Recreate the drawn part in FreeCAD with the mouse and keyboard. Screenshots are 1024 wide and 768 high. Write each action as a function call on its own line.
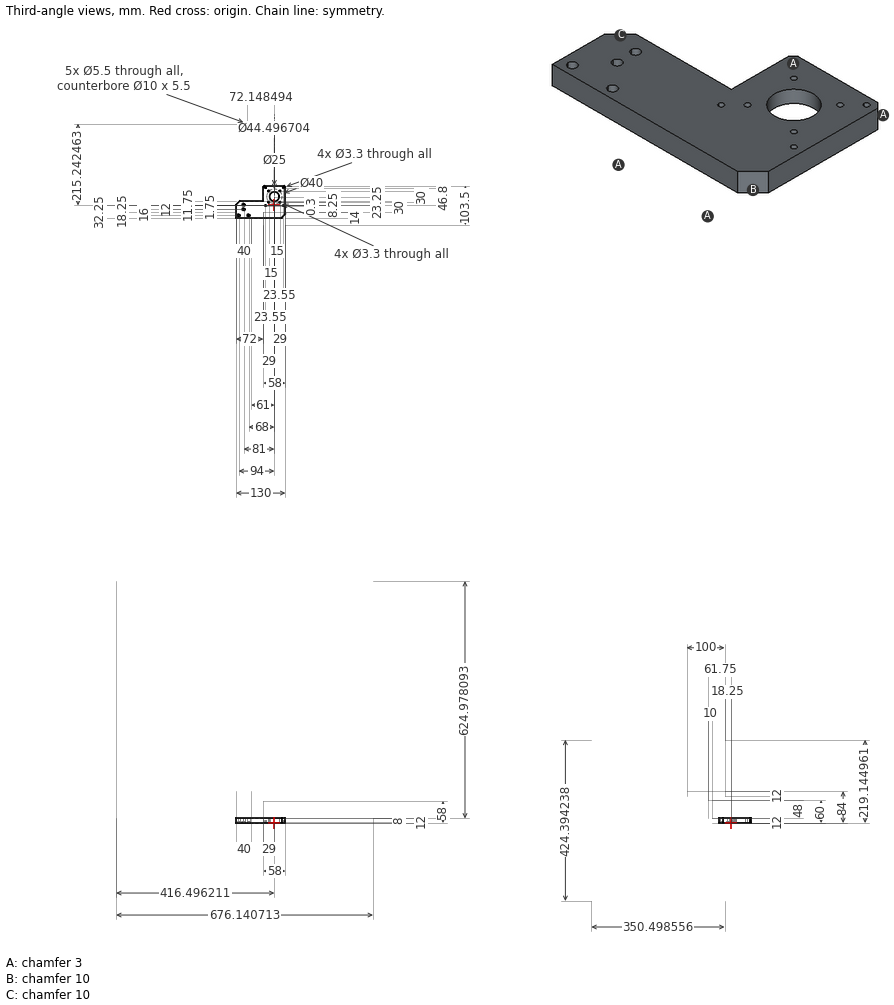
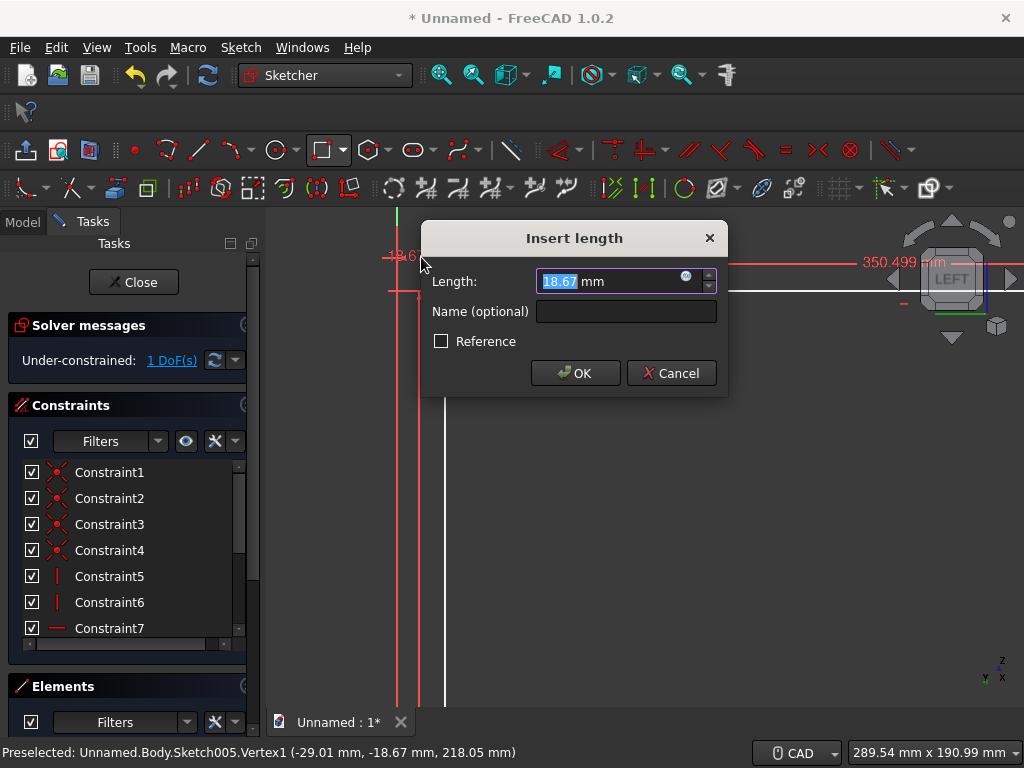
text(18.25)
key(Return)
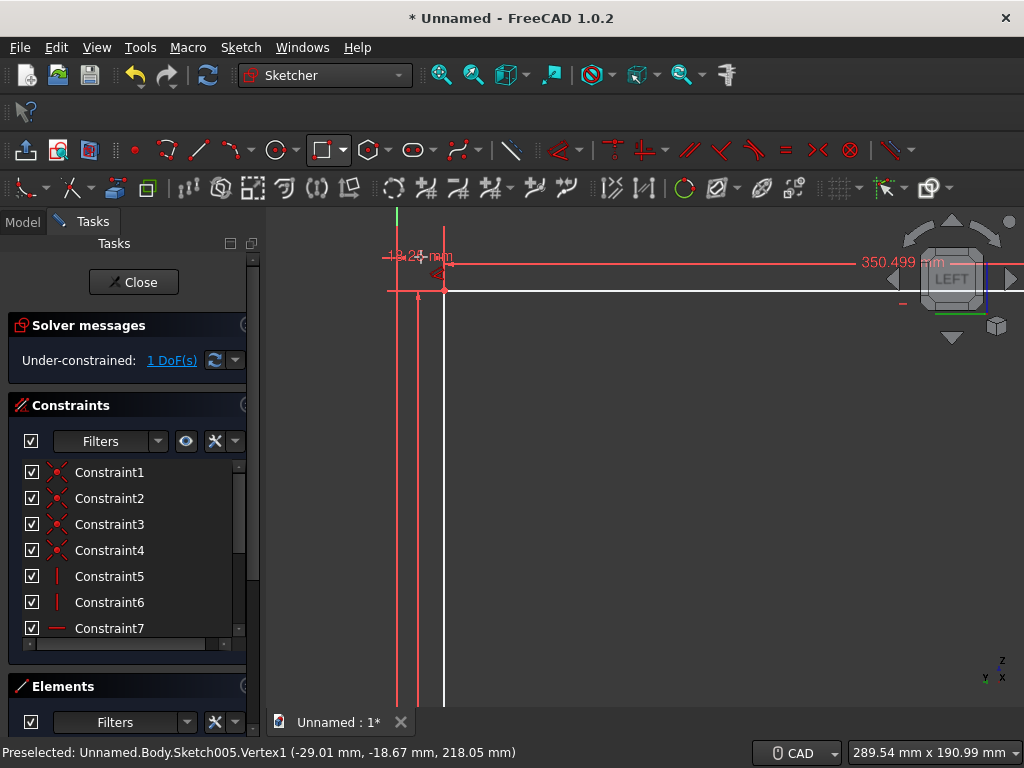
click(444, 291)
click(363, 485)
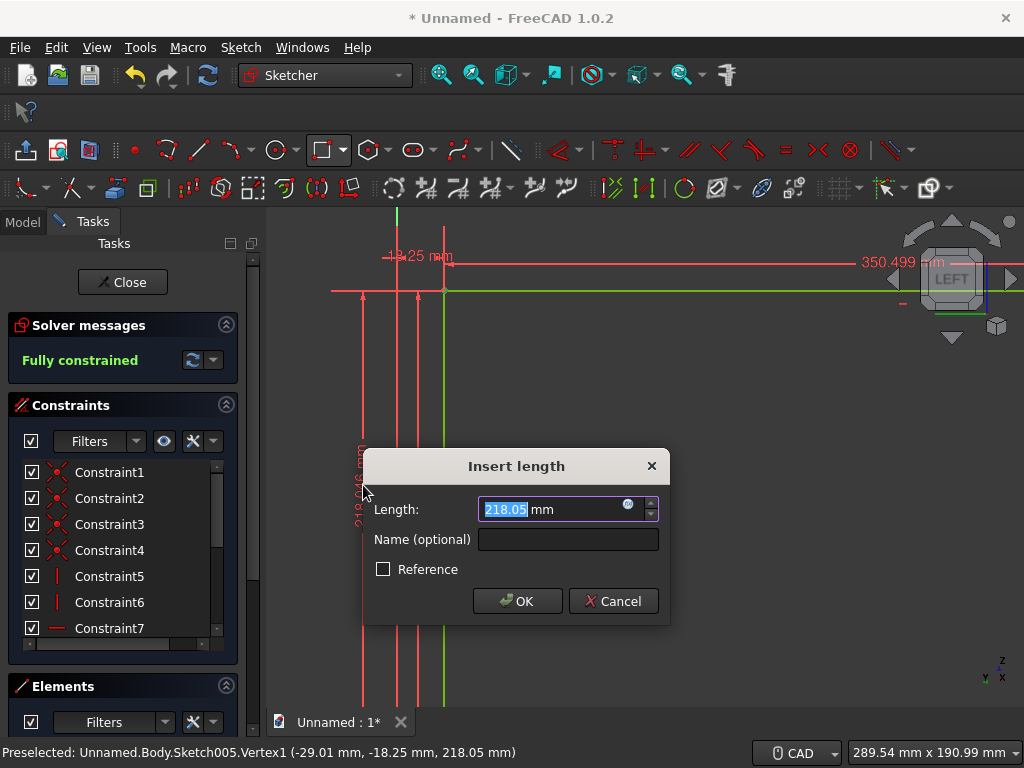
text(219.144961)
key(Return)
key(Escape)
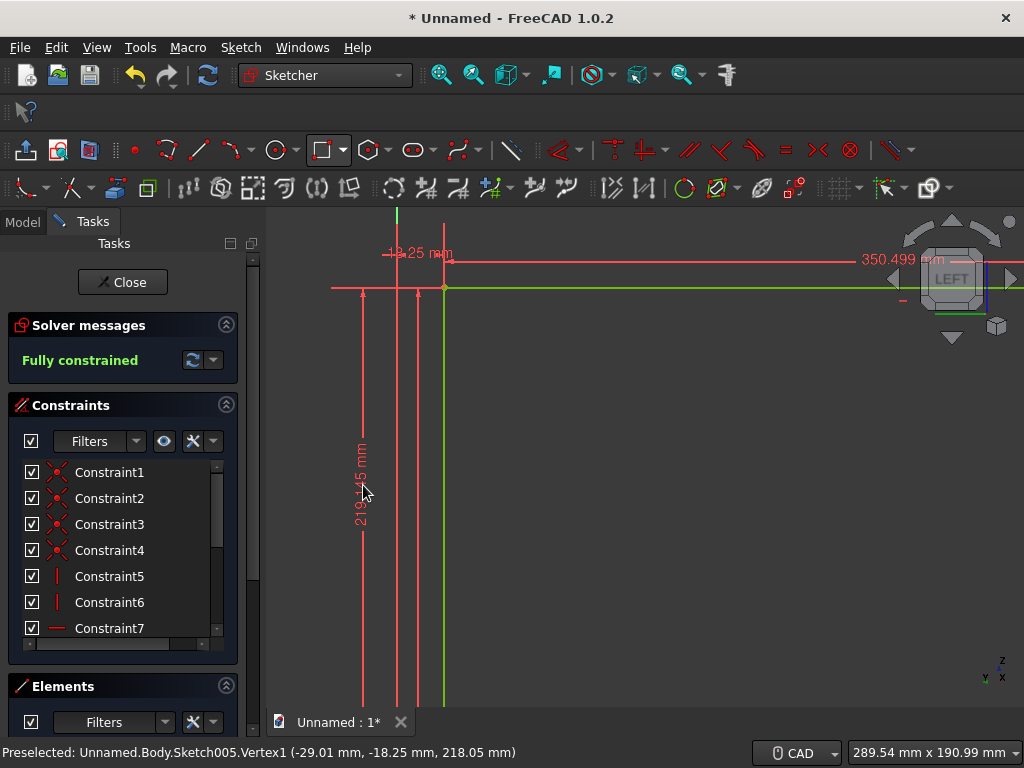
click(123, 282)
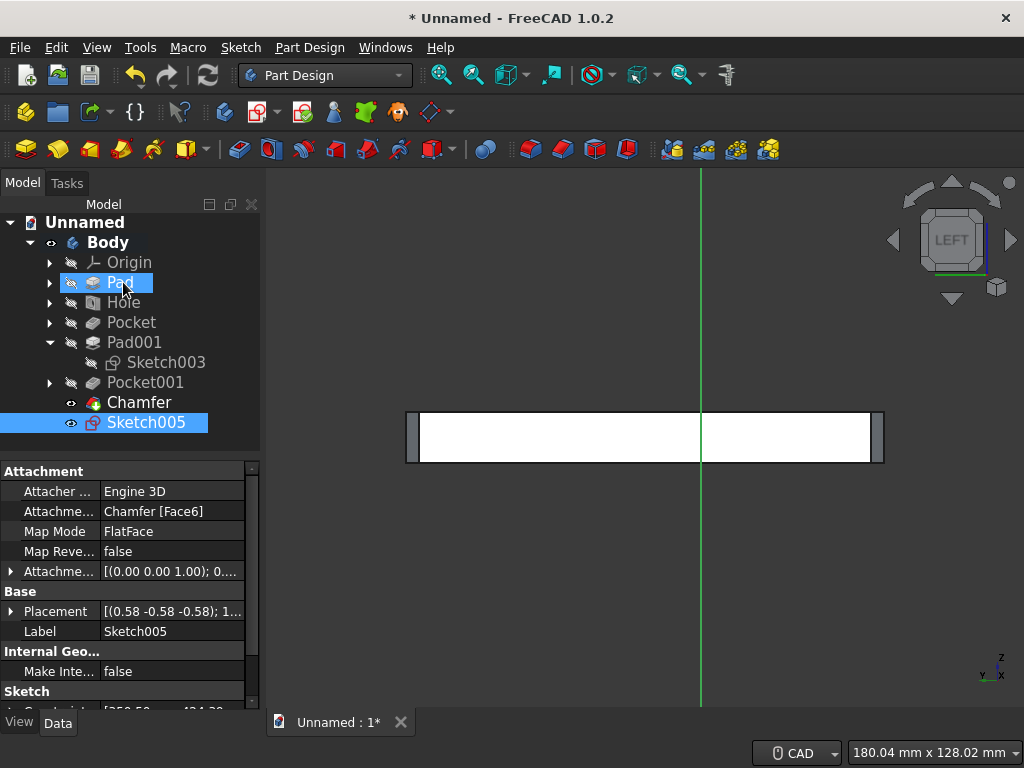
click(240, 150)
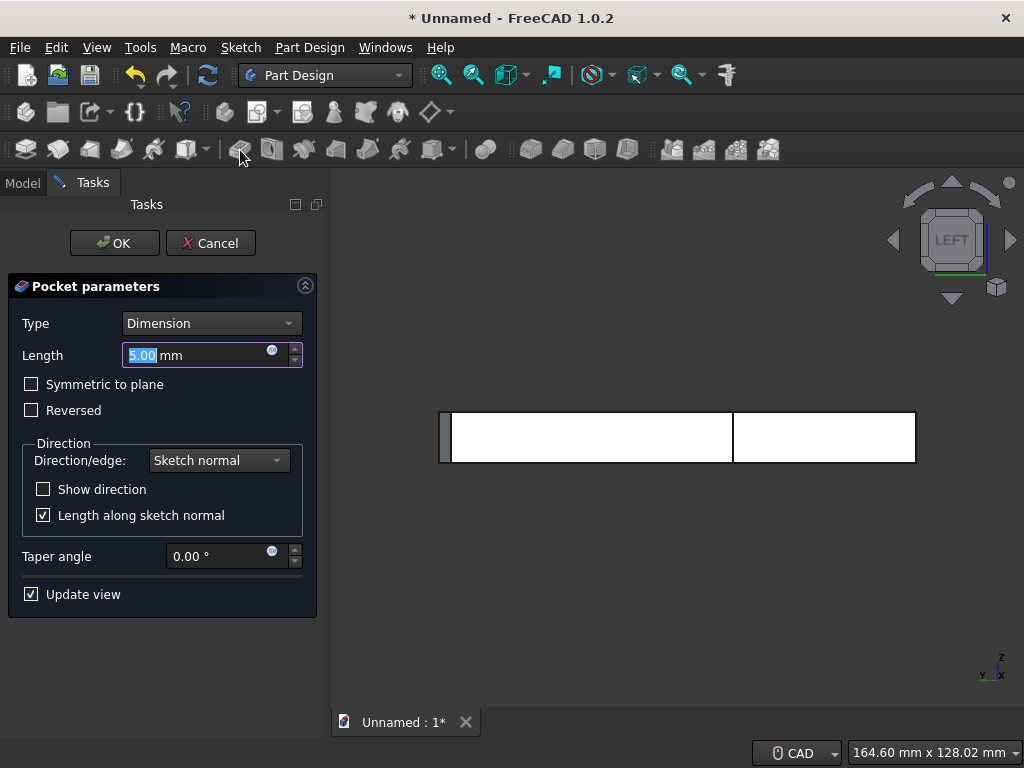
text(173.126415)
key(Tab)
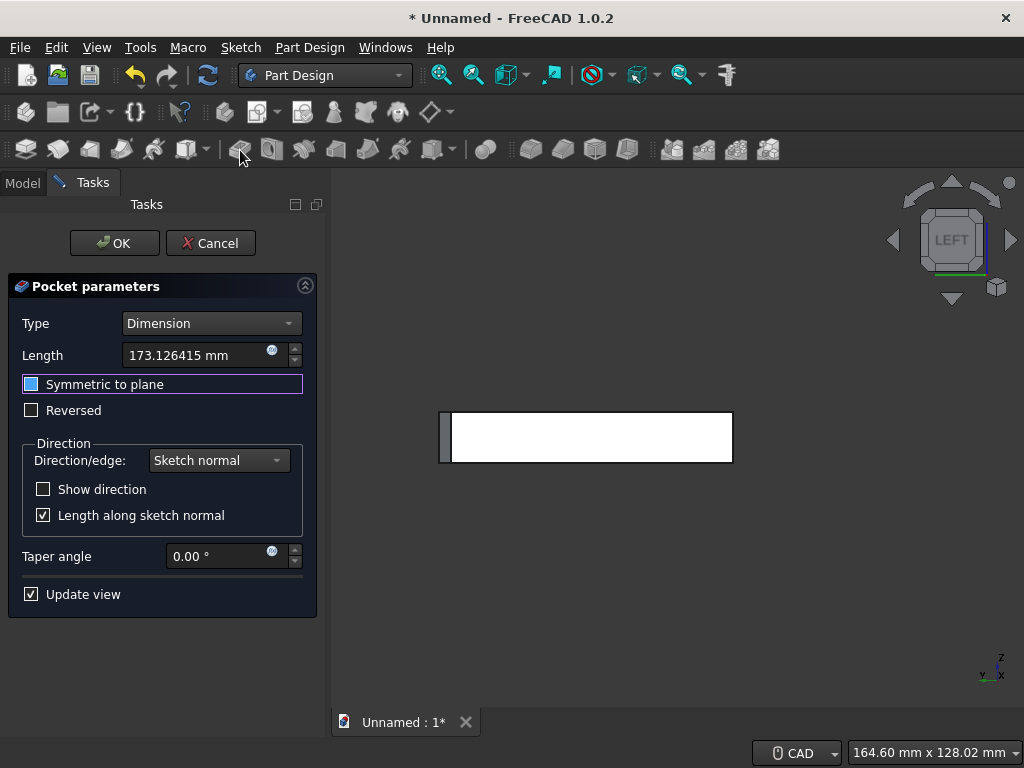
click(30, 384)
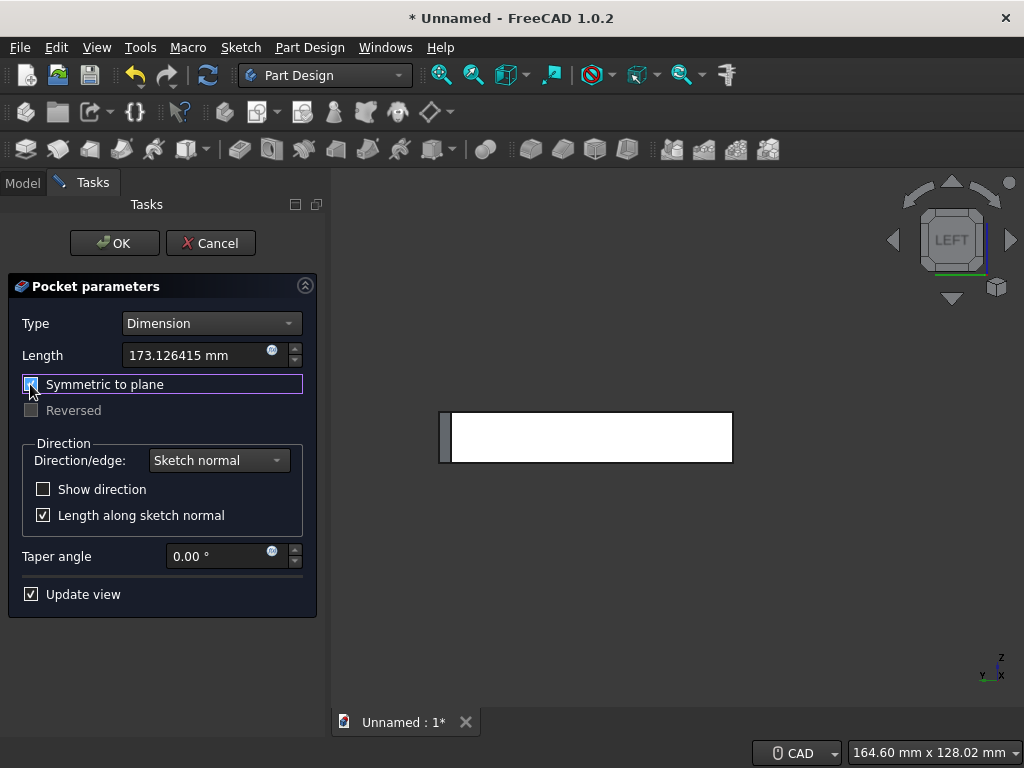
click(115, 243)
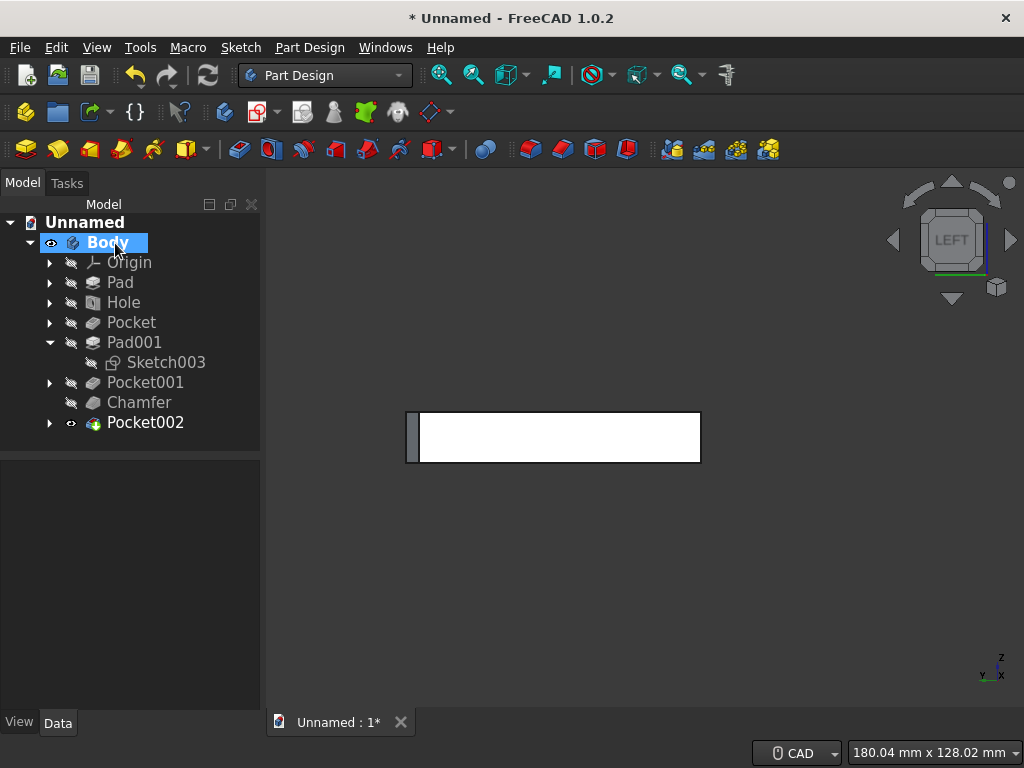
click(442, 76)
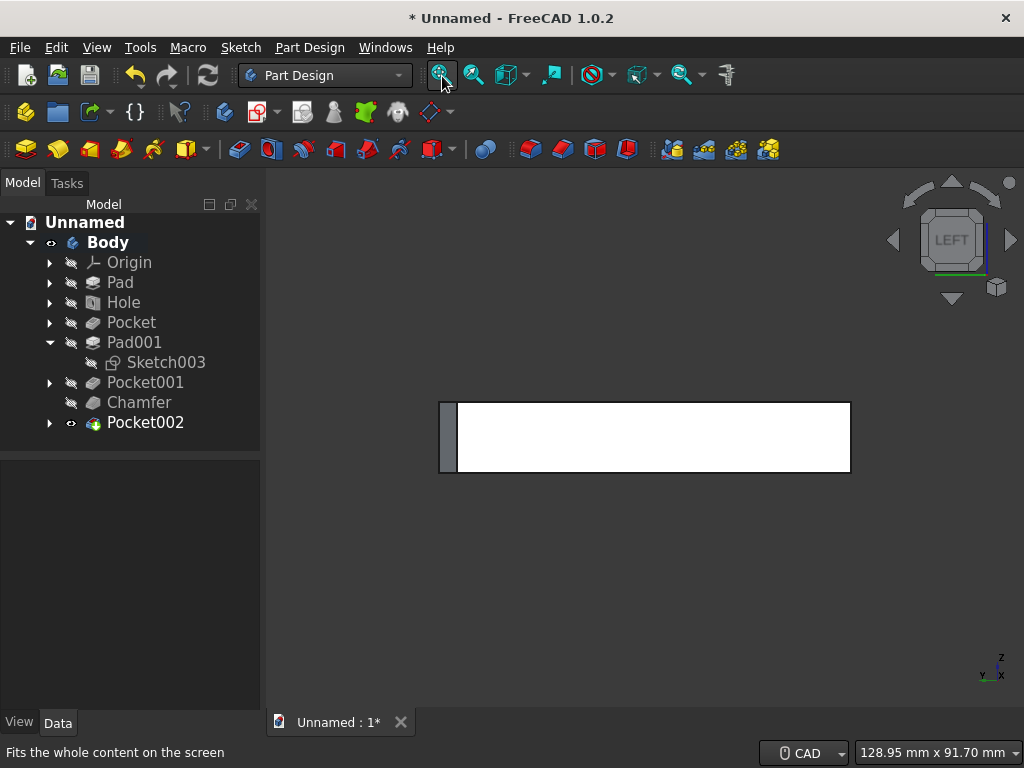
key(5)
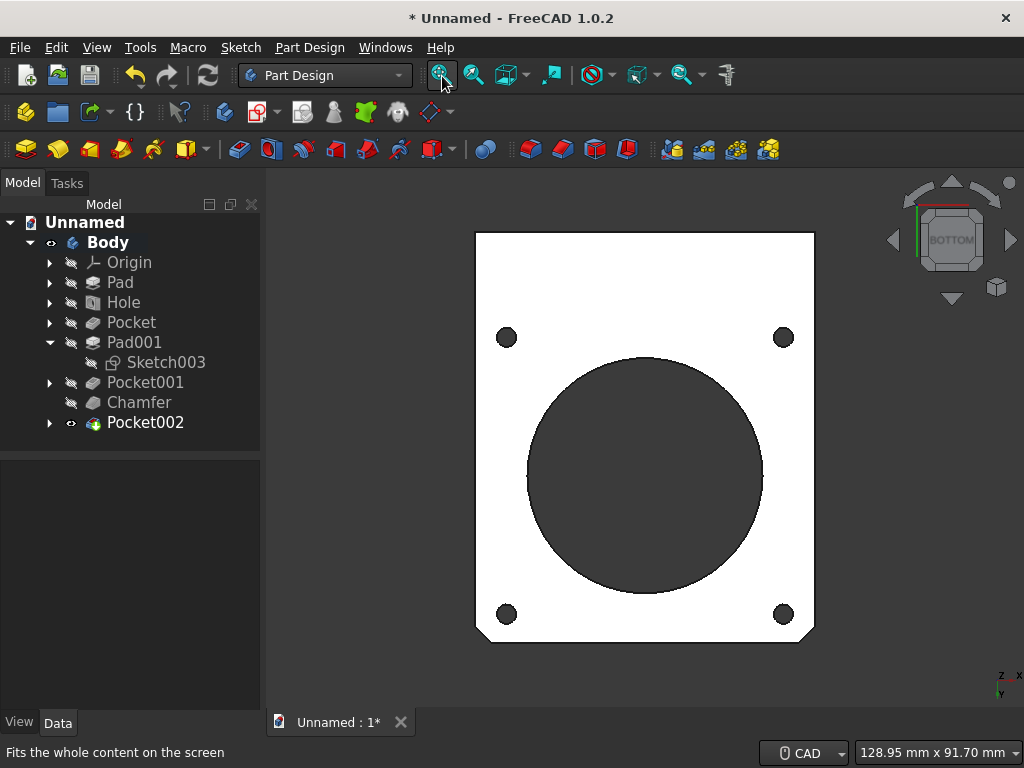
click(596, 319)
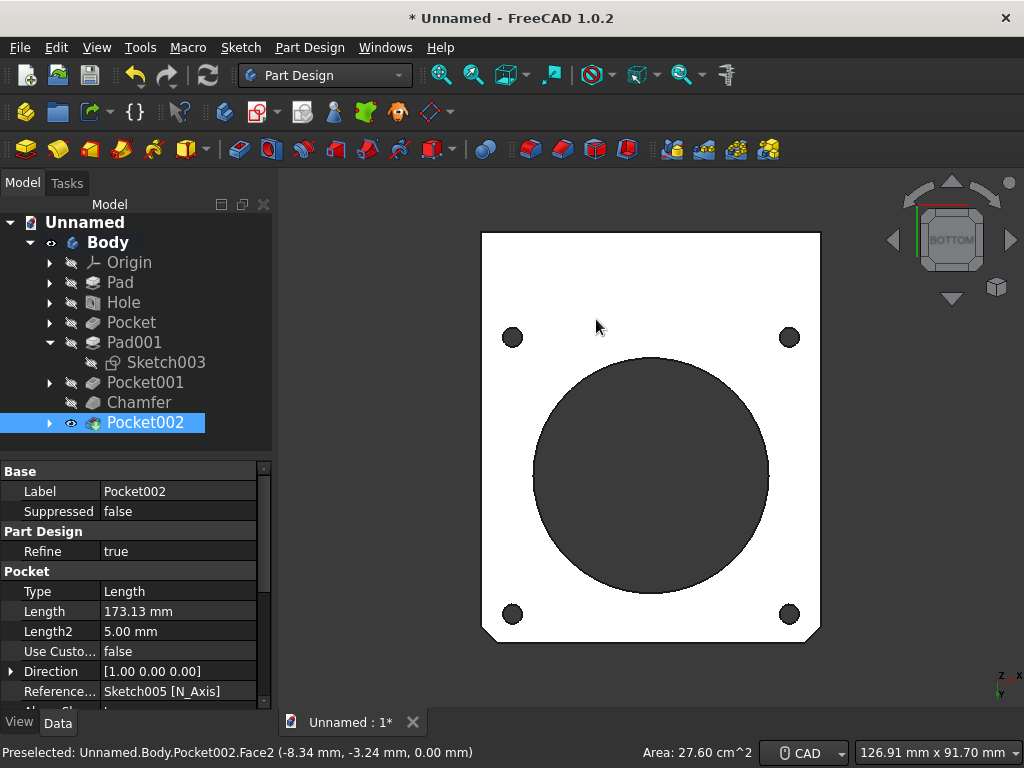
click(258, 112)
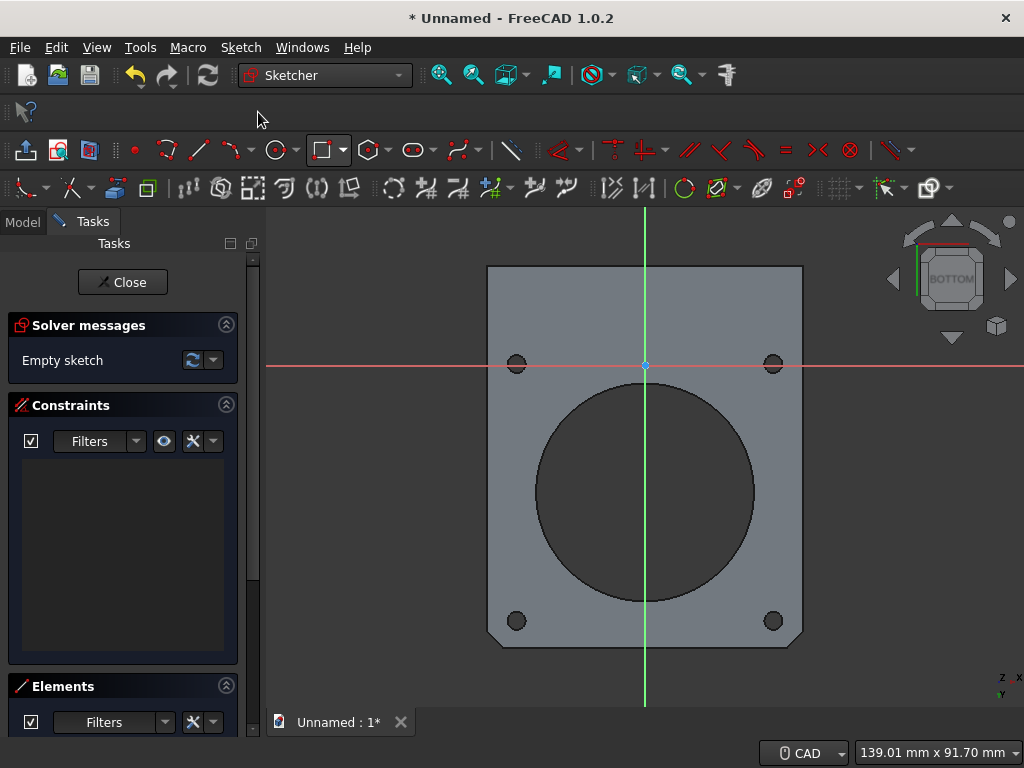
scroll(732, 675, down, 3)